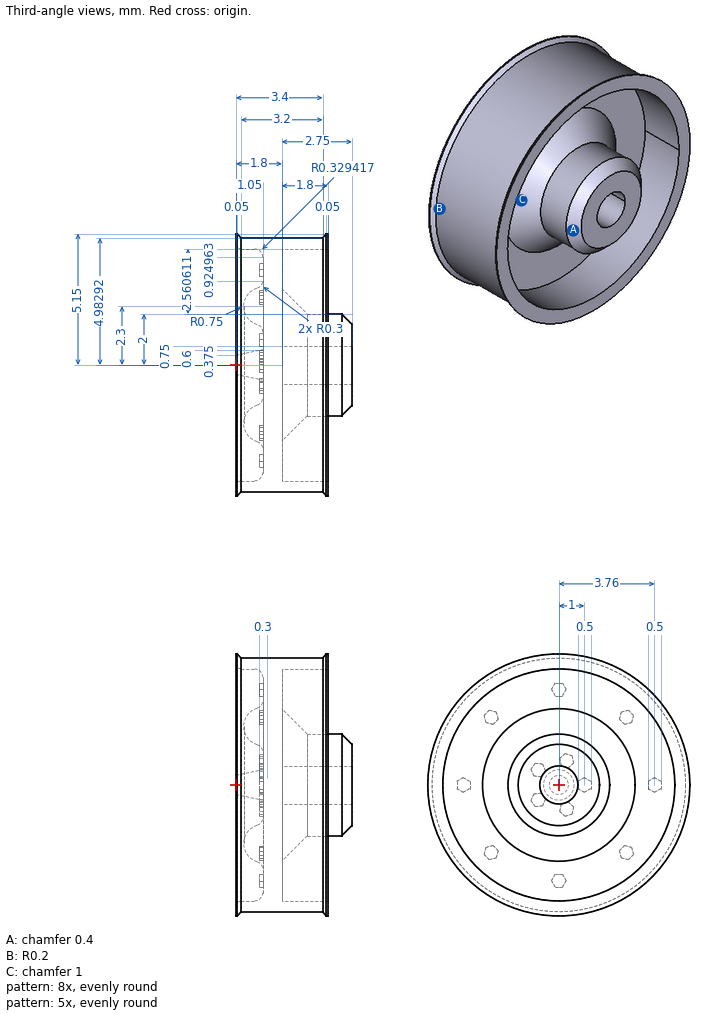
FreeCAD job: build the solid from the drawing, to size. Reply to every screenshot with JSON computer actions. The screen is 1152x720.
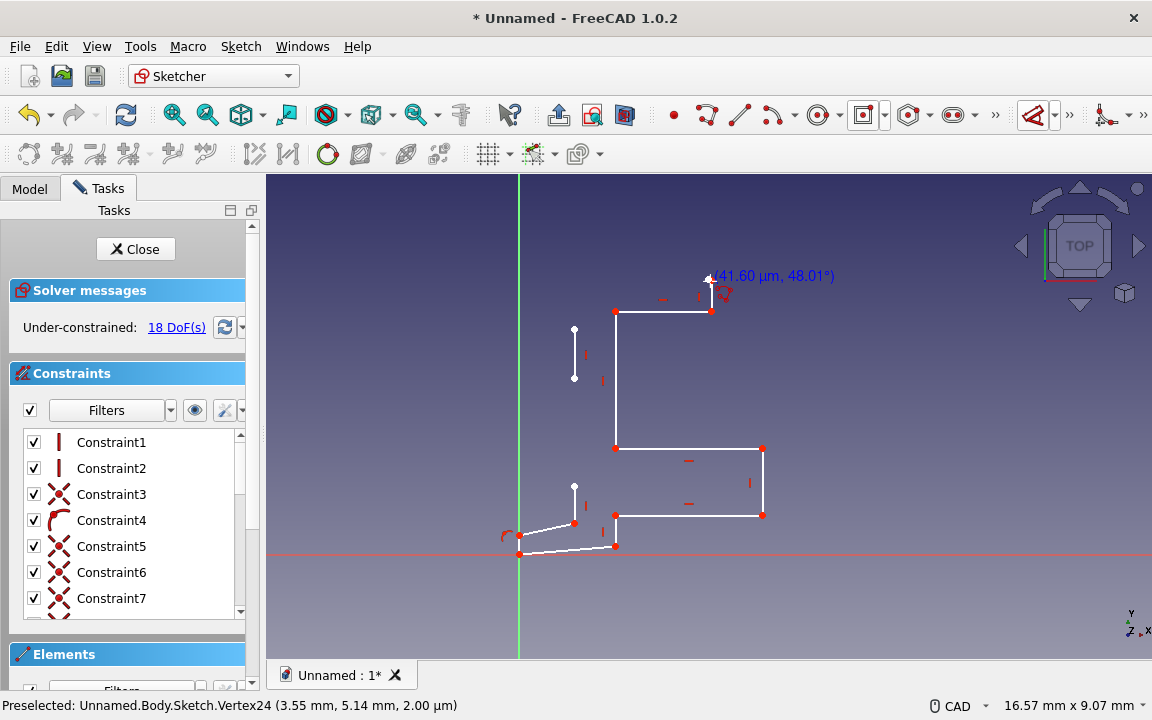
{"action": "scroll", "coordinate": [701, 288], "scroll_direction": "up", "scroll_amount": 2}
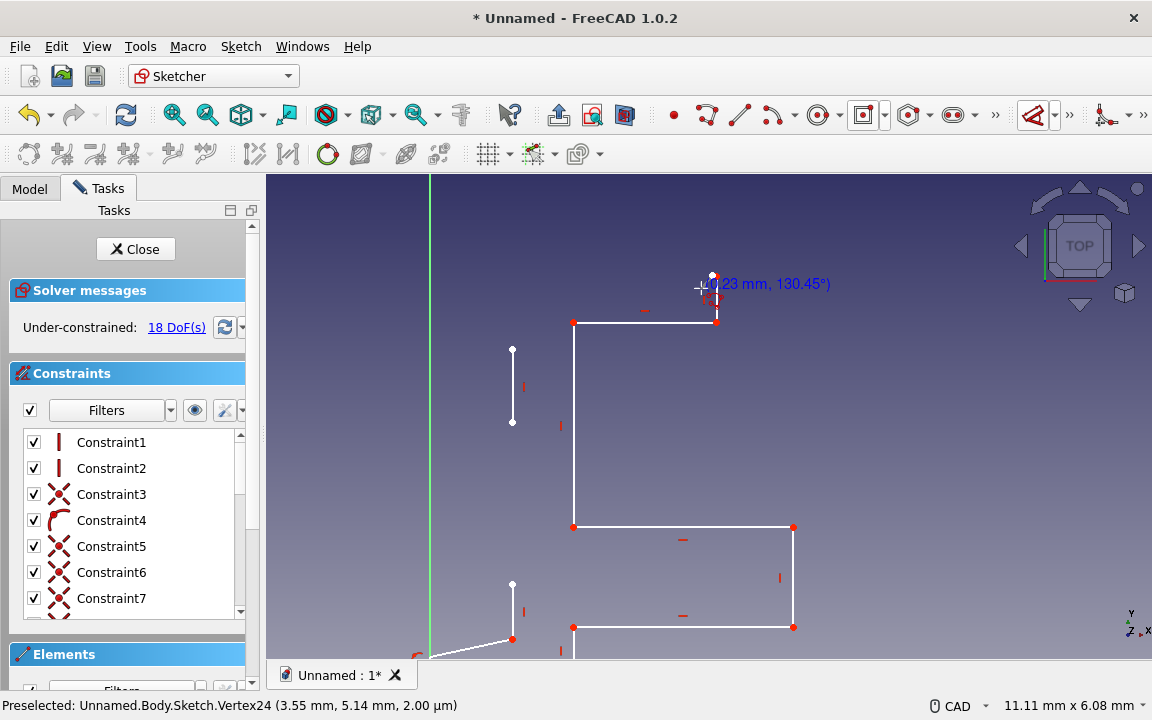
{"action": "left_click", "coordinate": [701, 288]}
{"action": "left_click", "coordinate": [445, 288]}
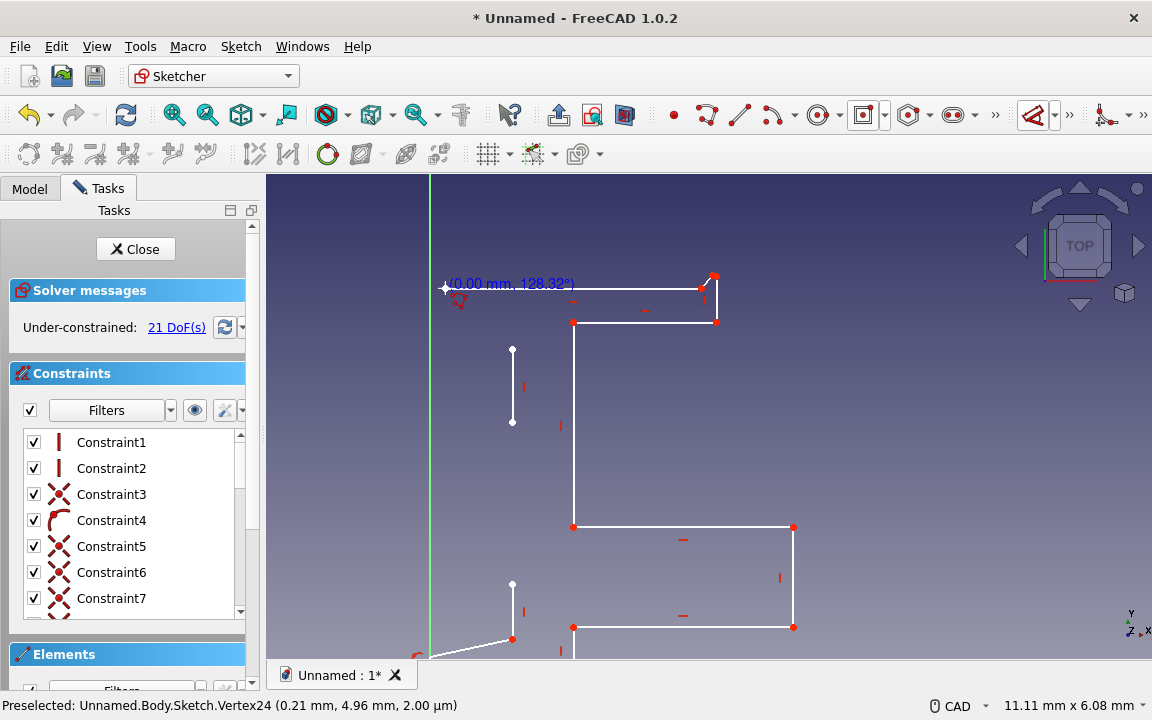
{"action": "scroll", "coordinate": [433, 275], "scroll_direction": "up", "scroll_amount": 7}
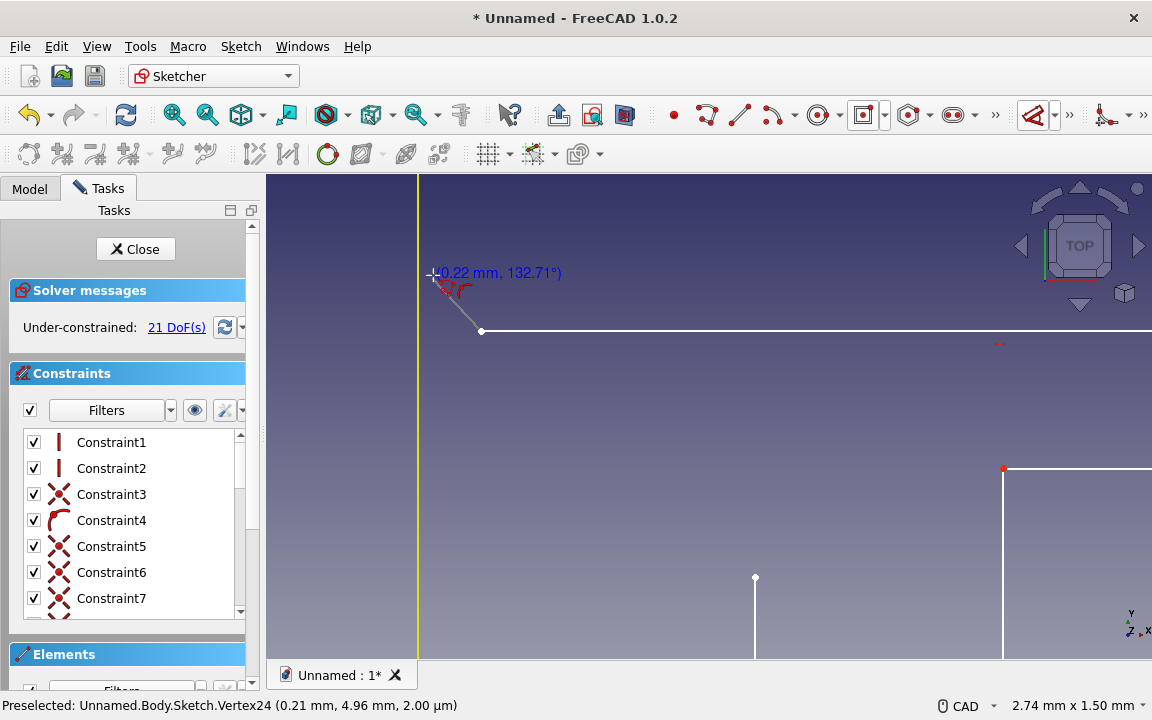
{"action": "left_click", "coordinate": [434, 274]}
{"action": "left_click", "coordinate": [418, 274]}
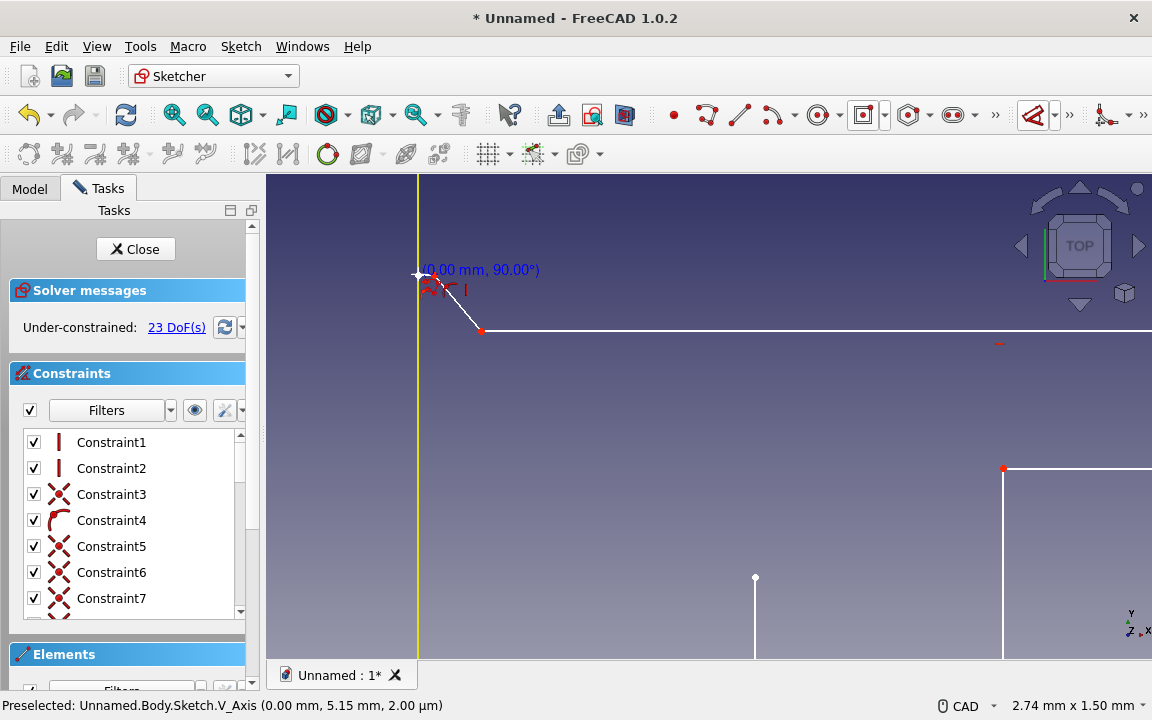
{"action": "scroll", "coordinate": [539, 280], "scroll_direction": "down", "scroll_amount": 9}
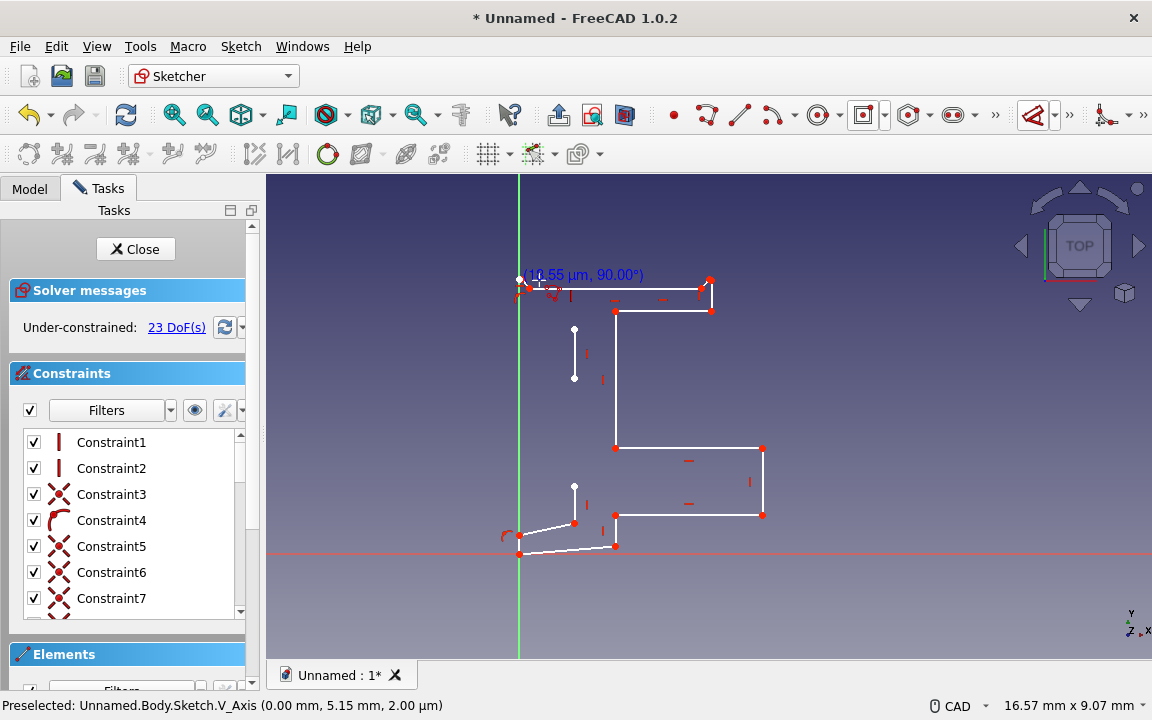
{"action": "left_click", "coordinate": [528, 311]}
{"action": "left_click", "coordinate": [558, 311]}
{"action": "right_click", "coordinate": [558, 311]}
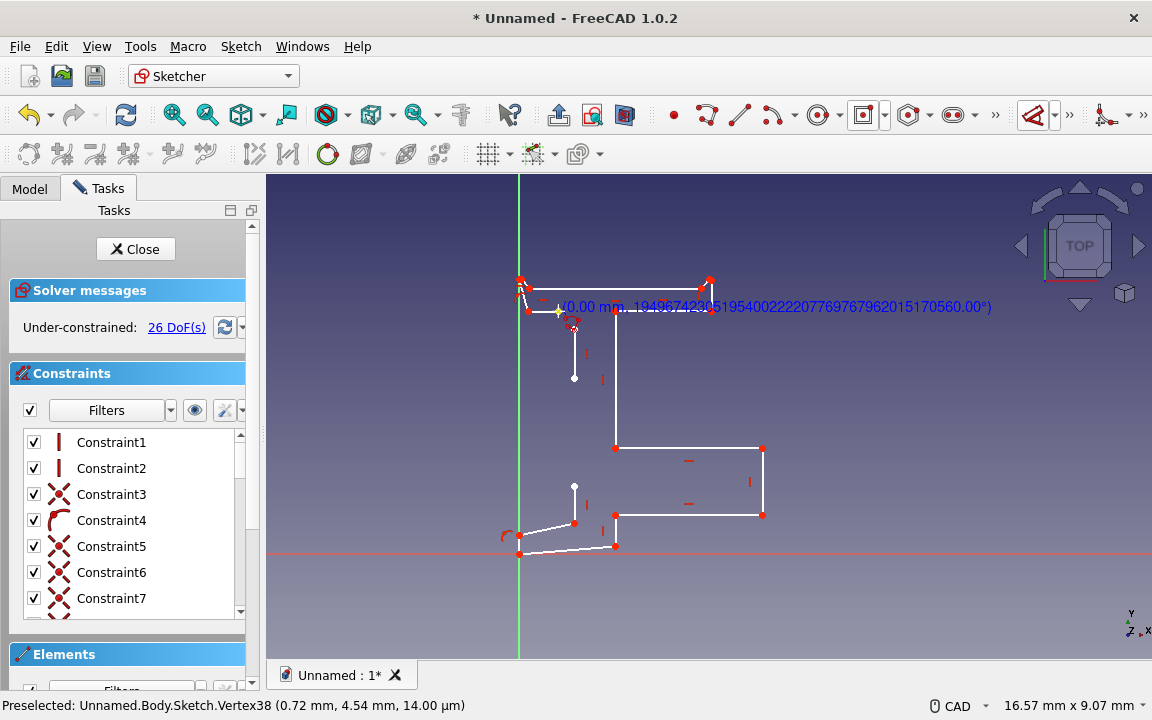
{"action": "left_click", "coordinate": [794, 116]}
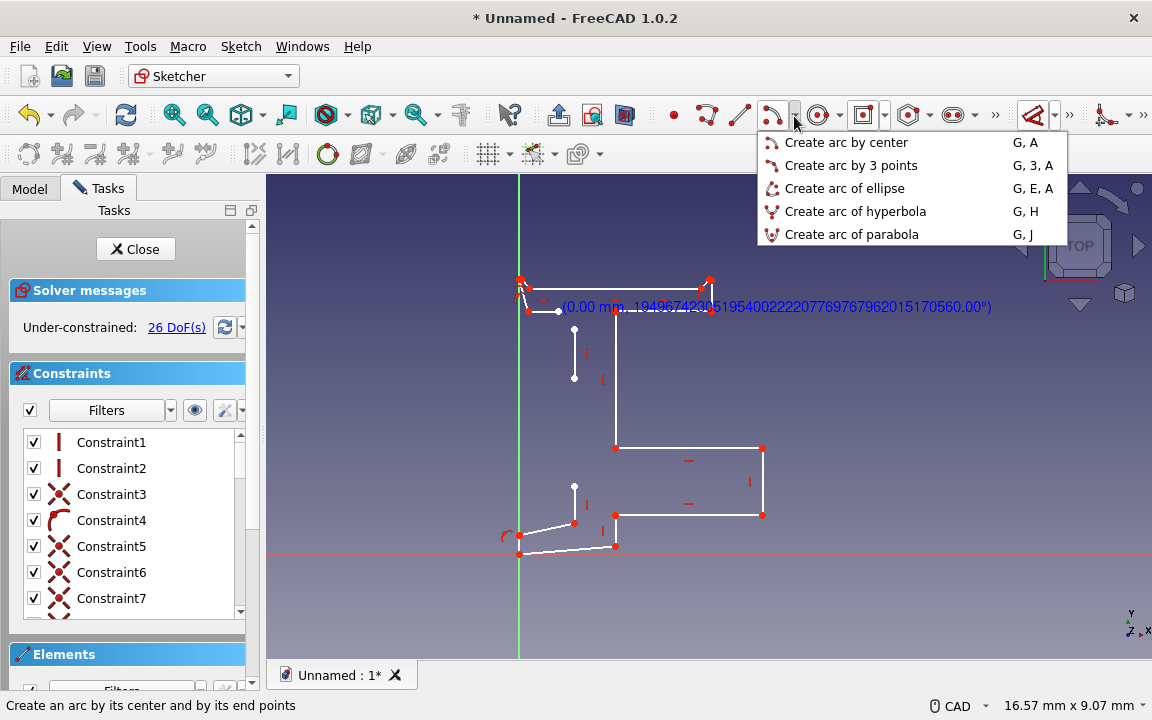
{"action": "left_click", "coordinate": [912, 166]}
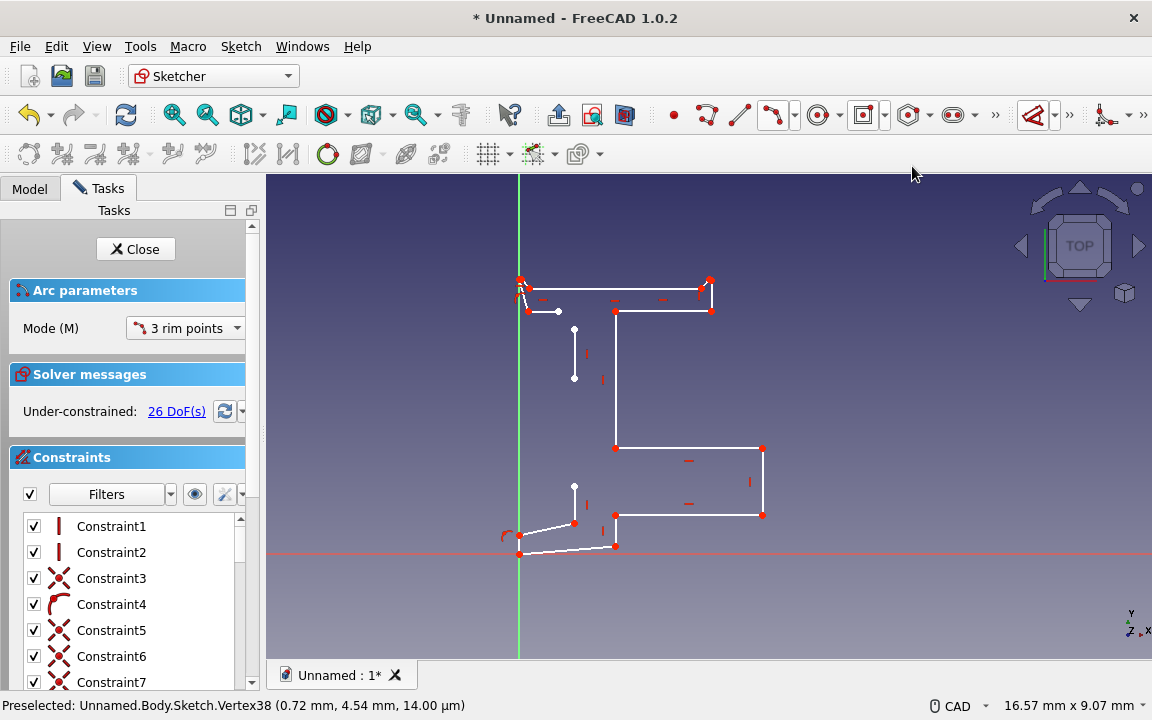
{"action": "left_click", "coordinate": [575, 378]}
{"action": "left_click", "coordinate": [564, 393]}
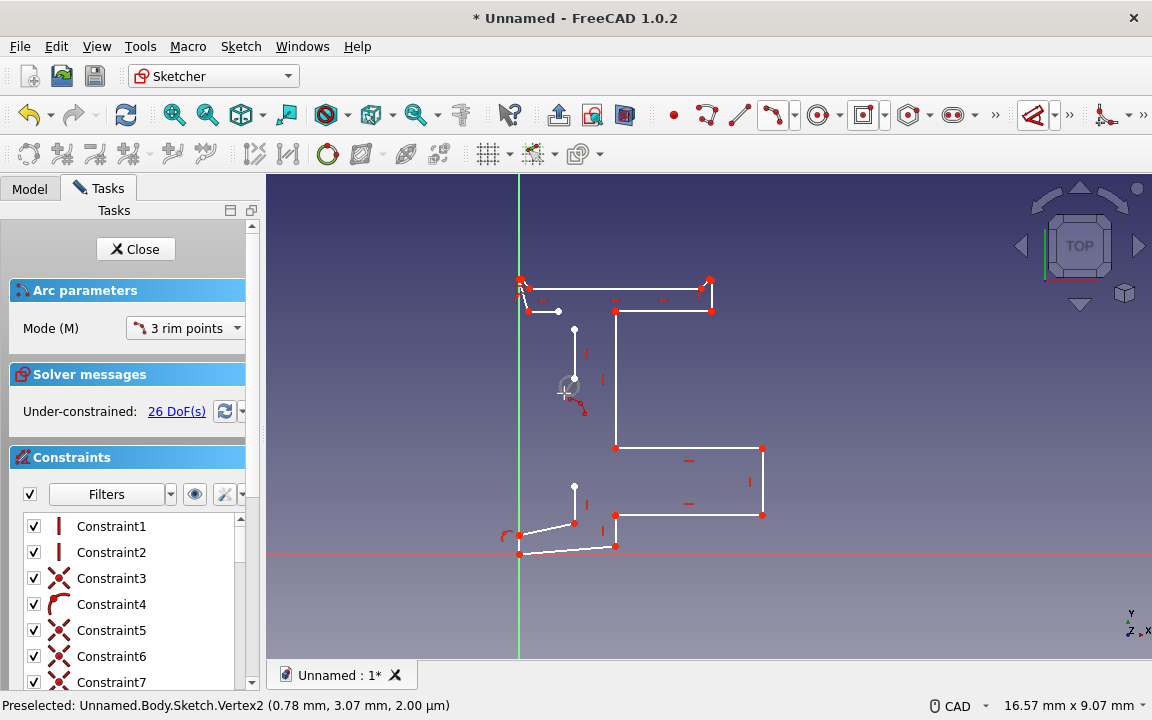
{"action": "scroll", "coordinate": [572, 387], "scroll_direction": "up", "scroll_amount": 9}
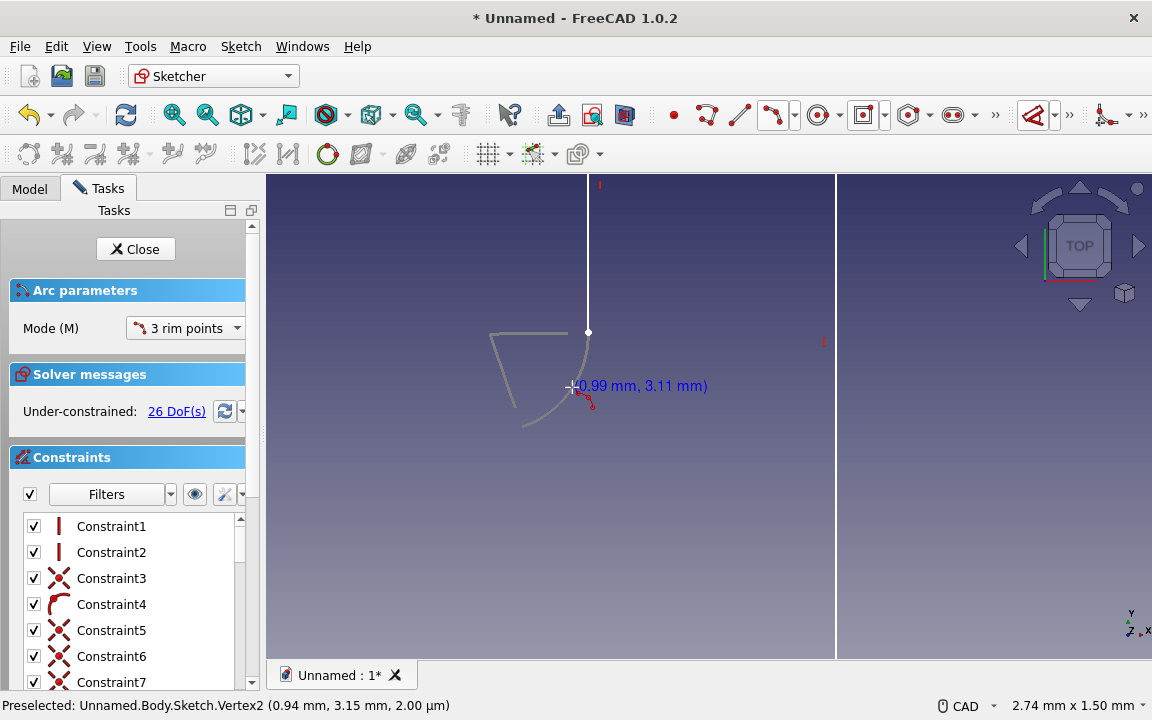
{"action": "left_click", "coordinate": [572, 387]}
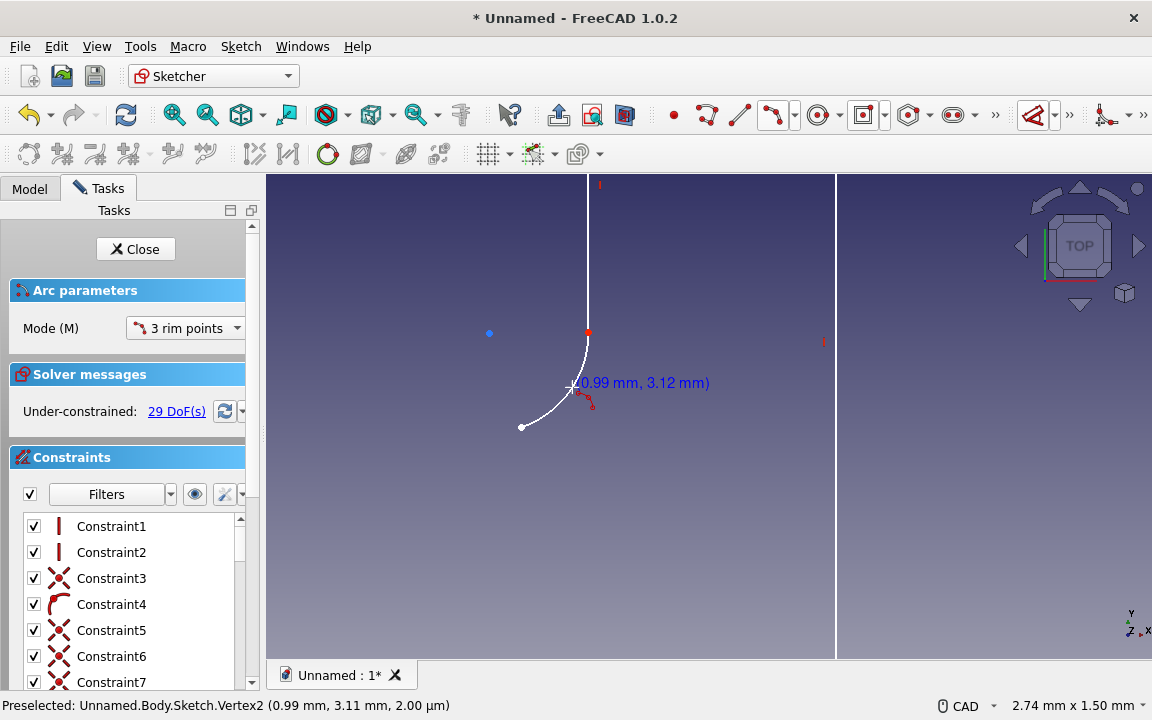
{"action": "scroll", "coordinate": [572, 387], "scroll_direction": "down", "scroll_amount": 9}